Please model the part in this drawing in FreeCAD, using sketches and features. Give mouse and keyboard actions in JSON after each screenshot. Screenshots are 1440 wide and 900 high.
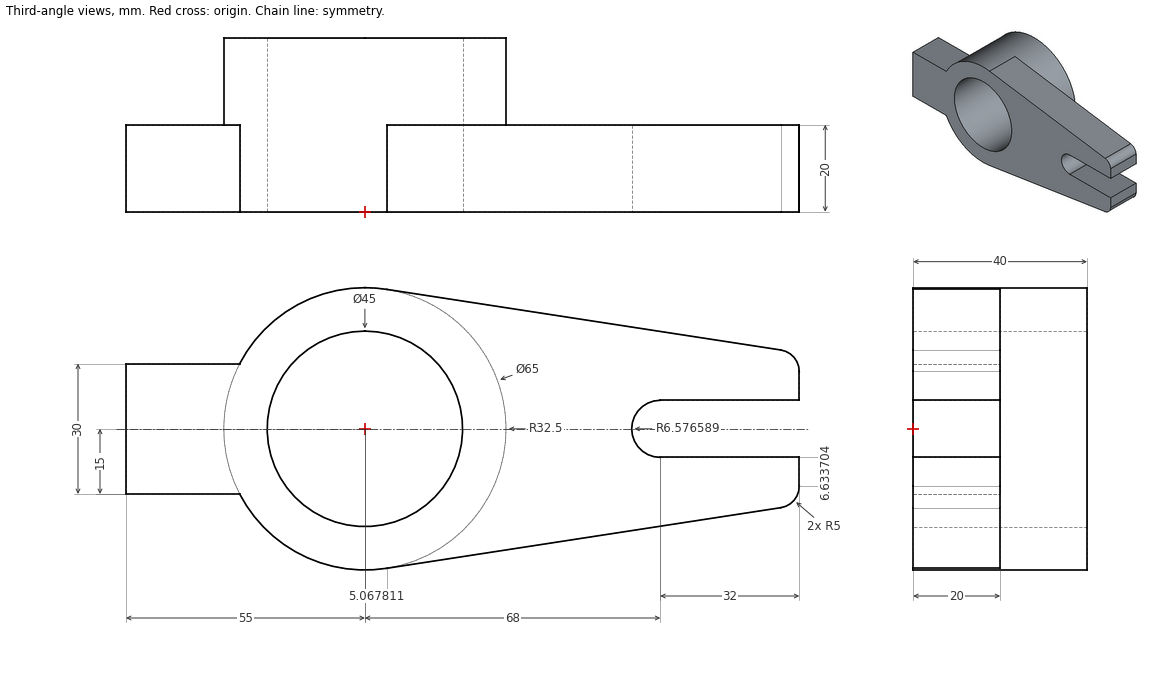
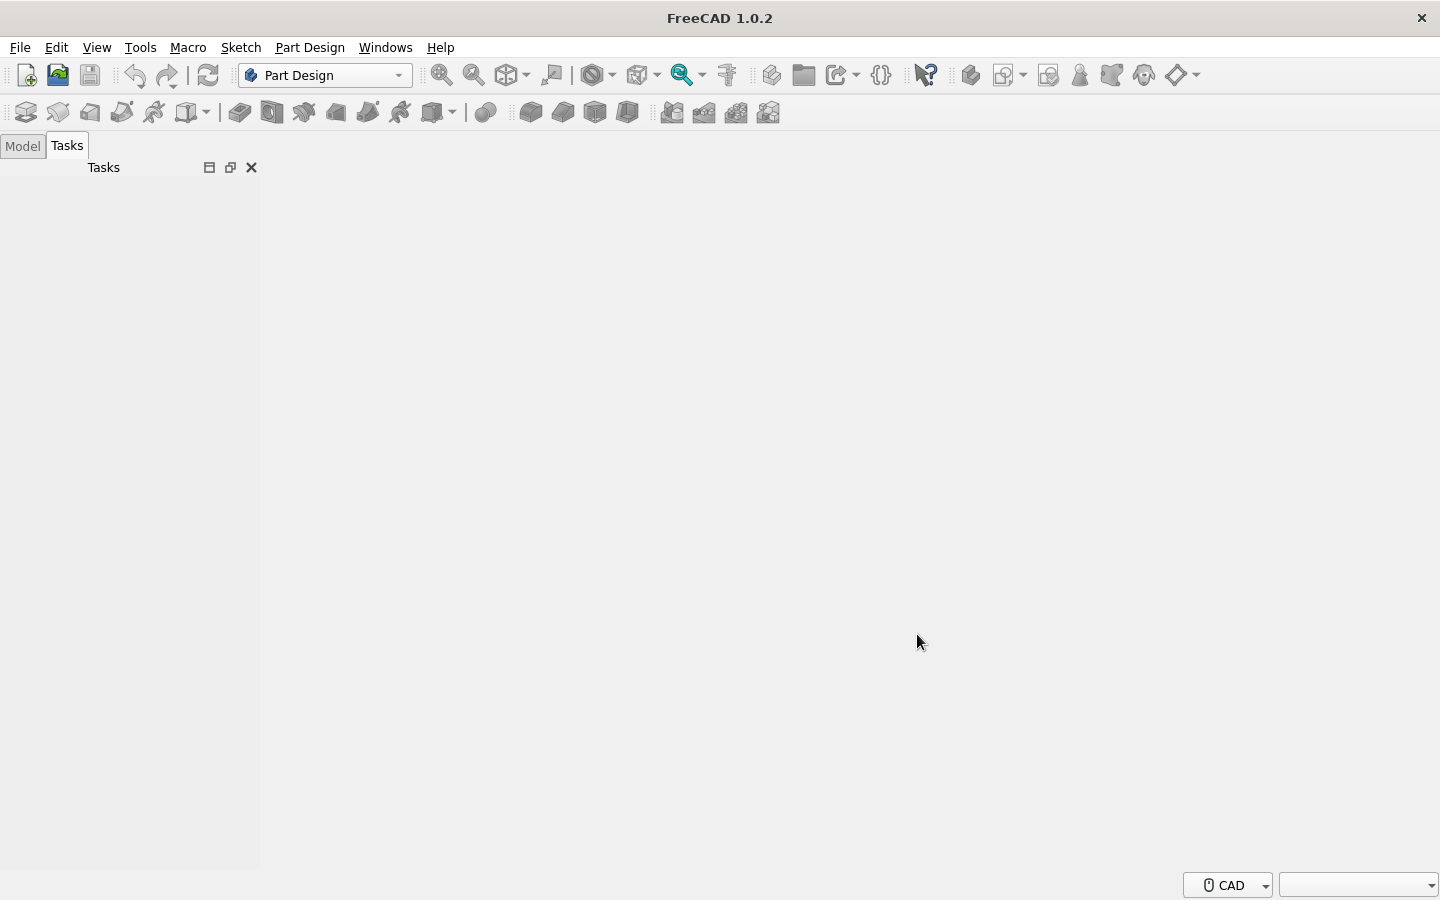
{"action": "left_click", "coordinate": [26, 76]}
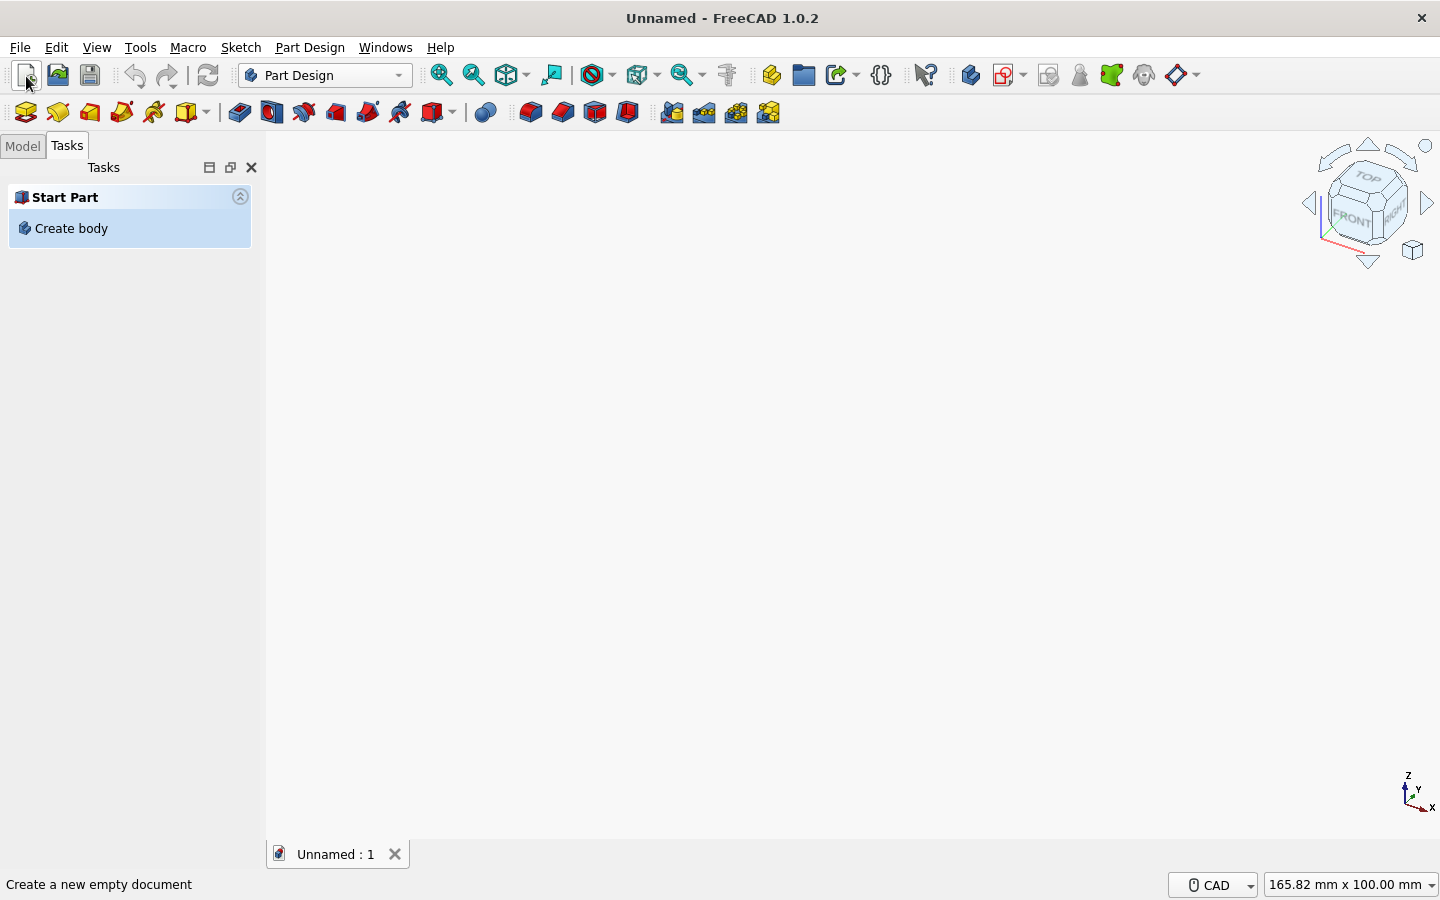
{"action": "left_click", "coordinate": [1004, 76]}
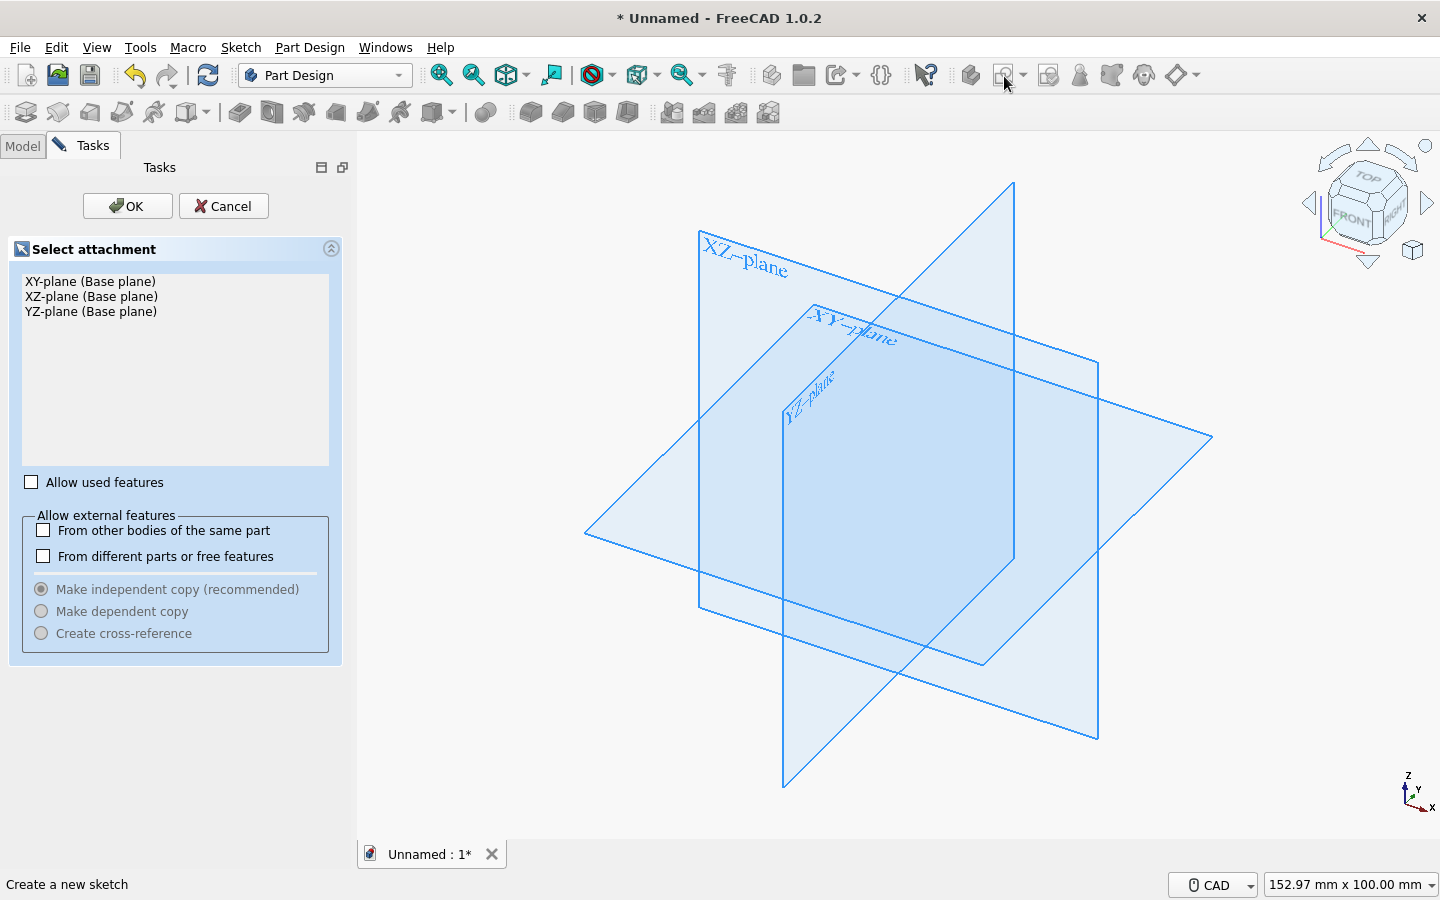
{"action": "left_click", "coordinate": [82, 296]}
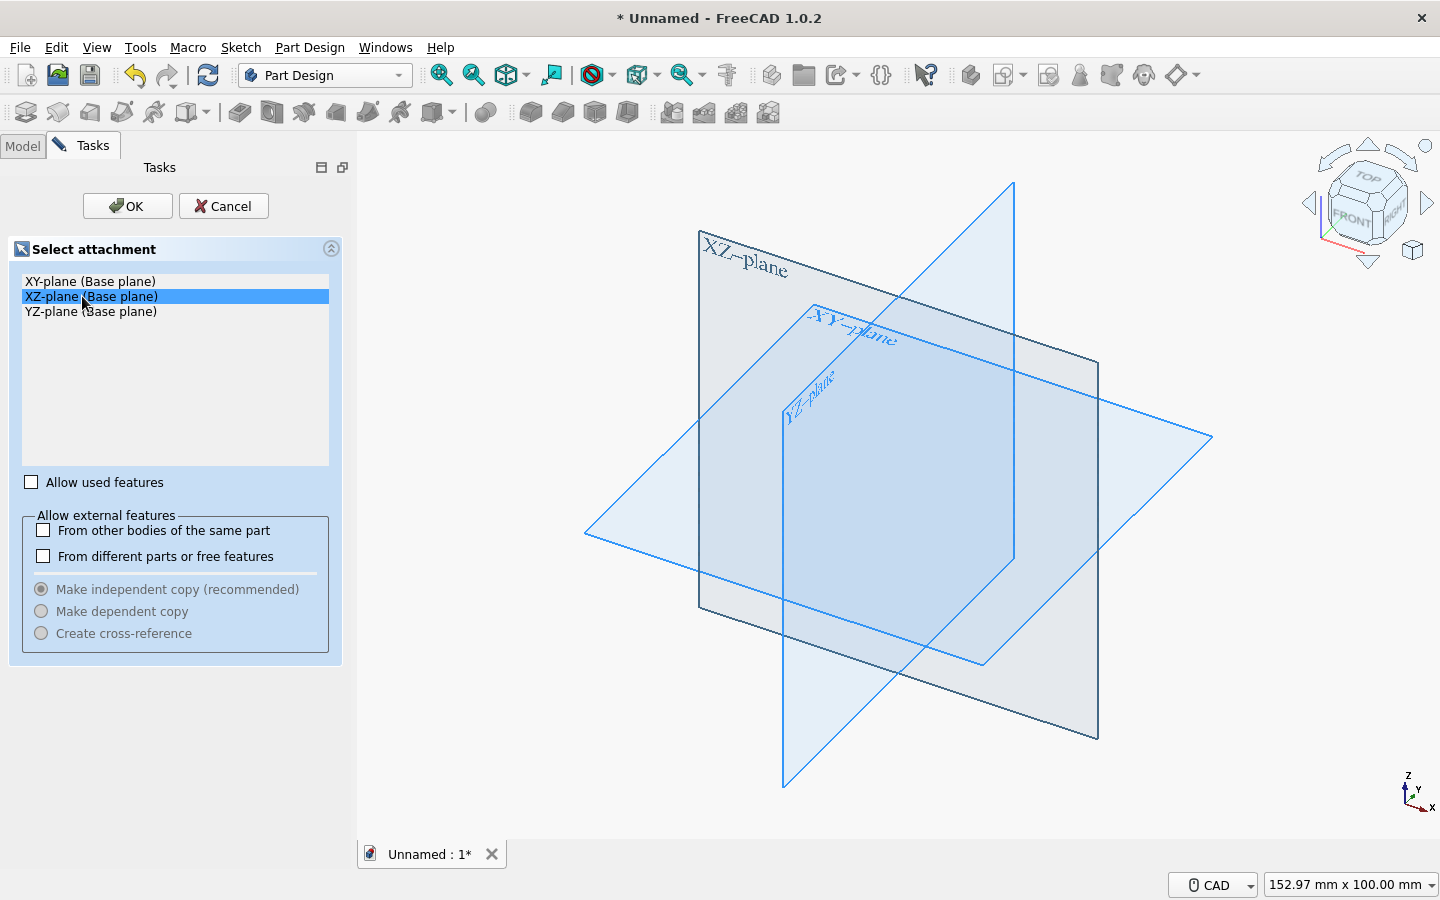
{"action": "left_click", "coordinate": [128, 206]}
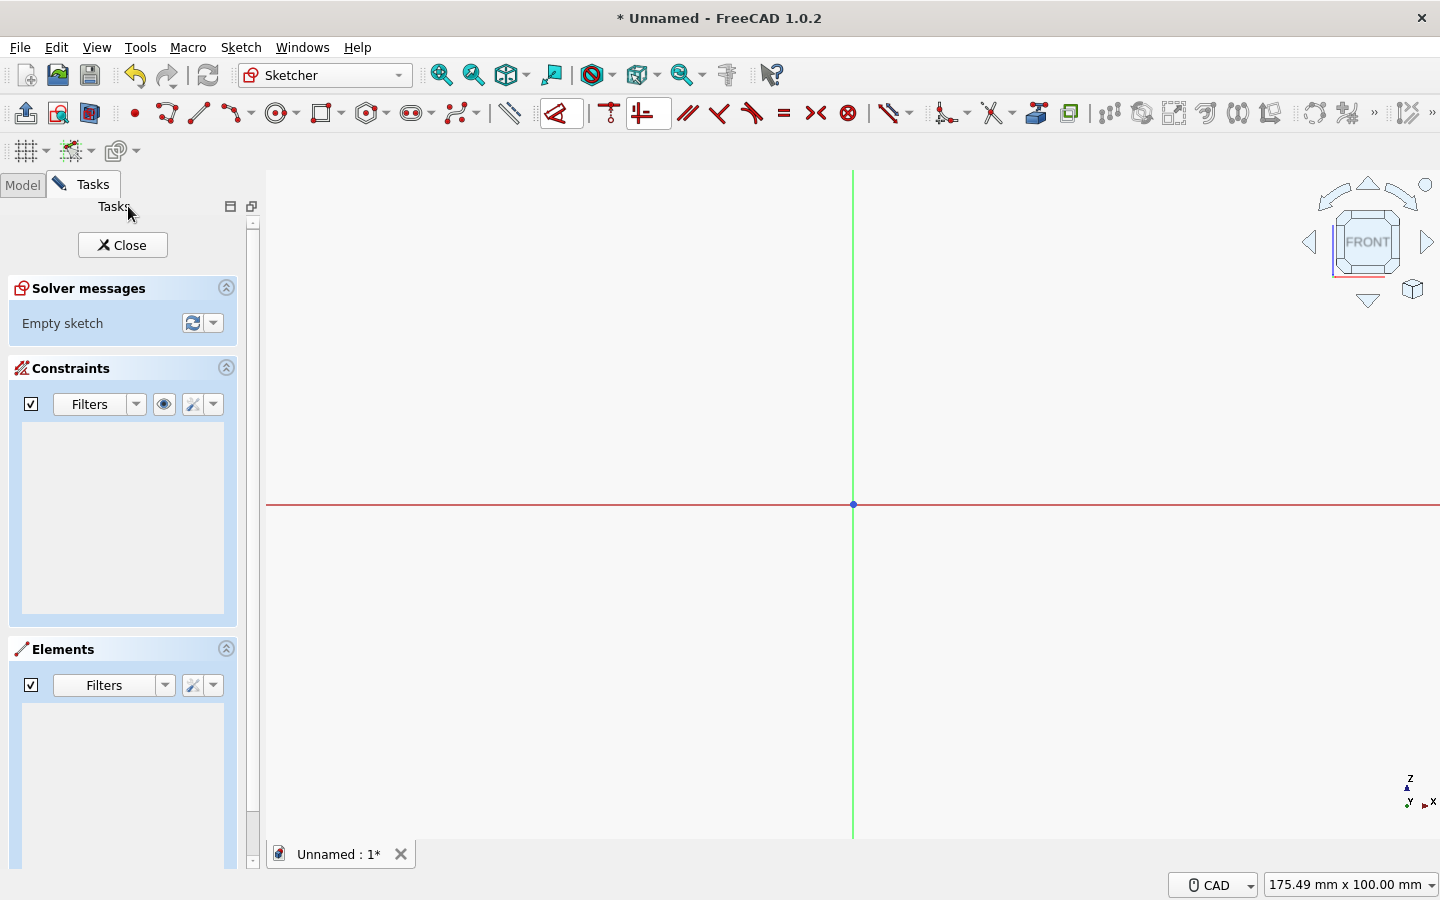
{"action": "left_click", "coordinate": [276, 114]}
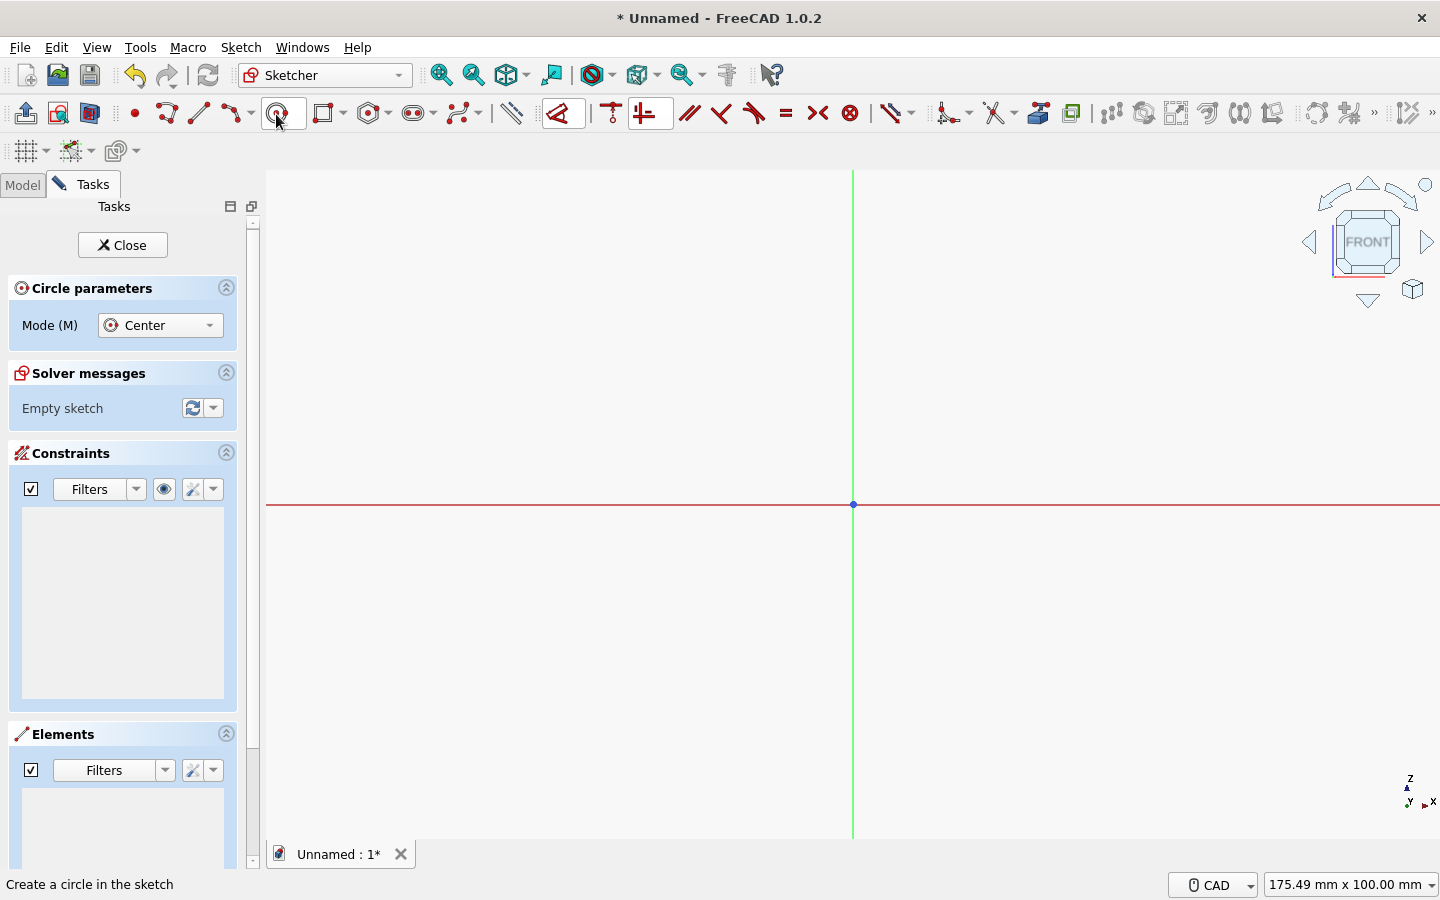
{"action": "left_click", "coordinate": [853, 504]}
{"action": "mouse_move", "coordinate": [1007, 351]}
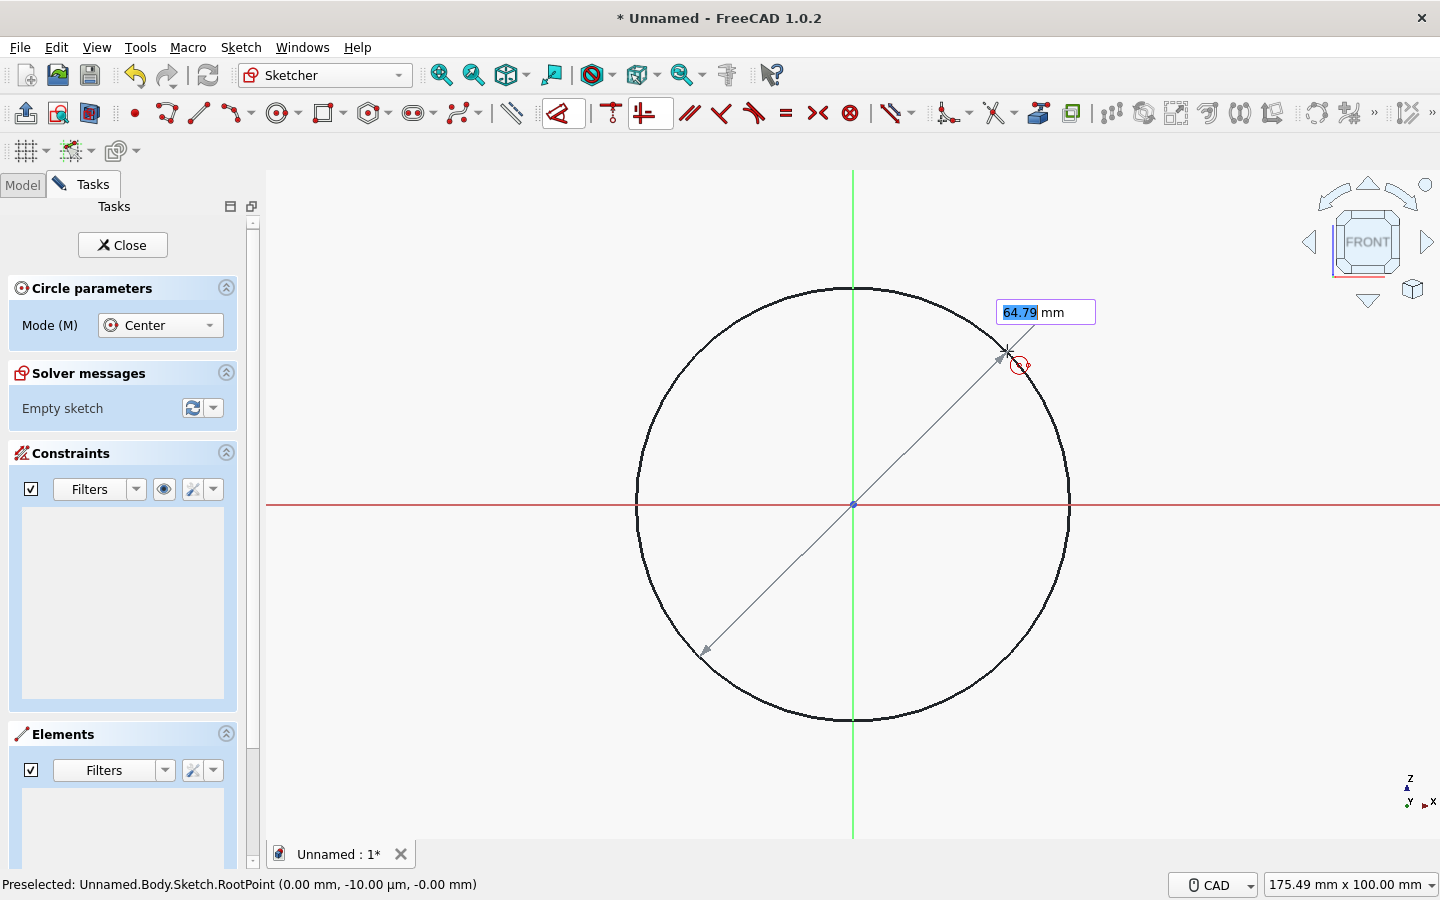
{"action": "type", "text": "65"}
{"action": "key", "text": "Return"}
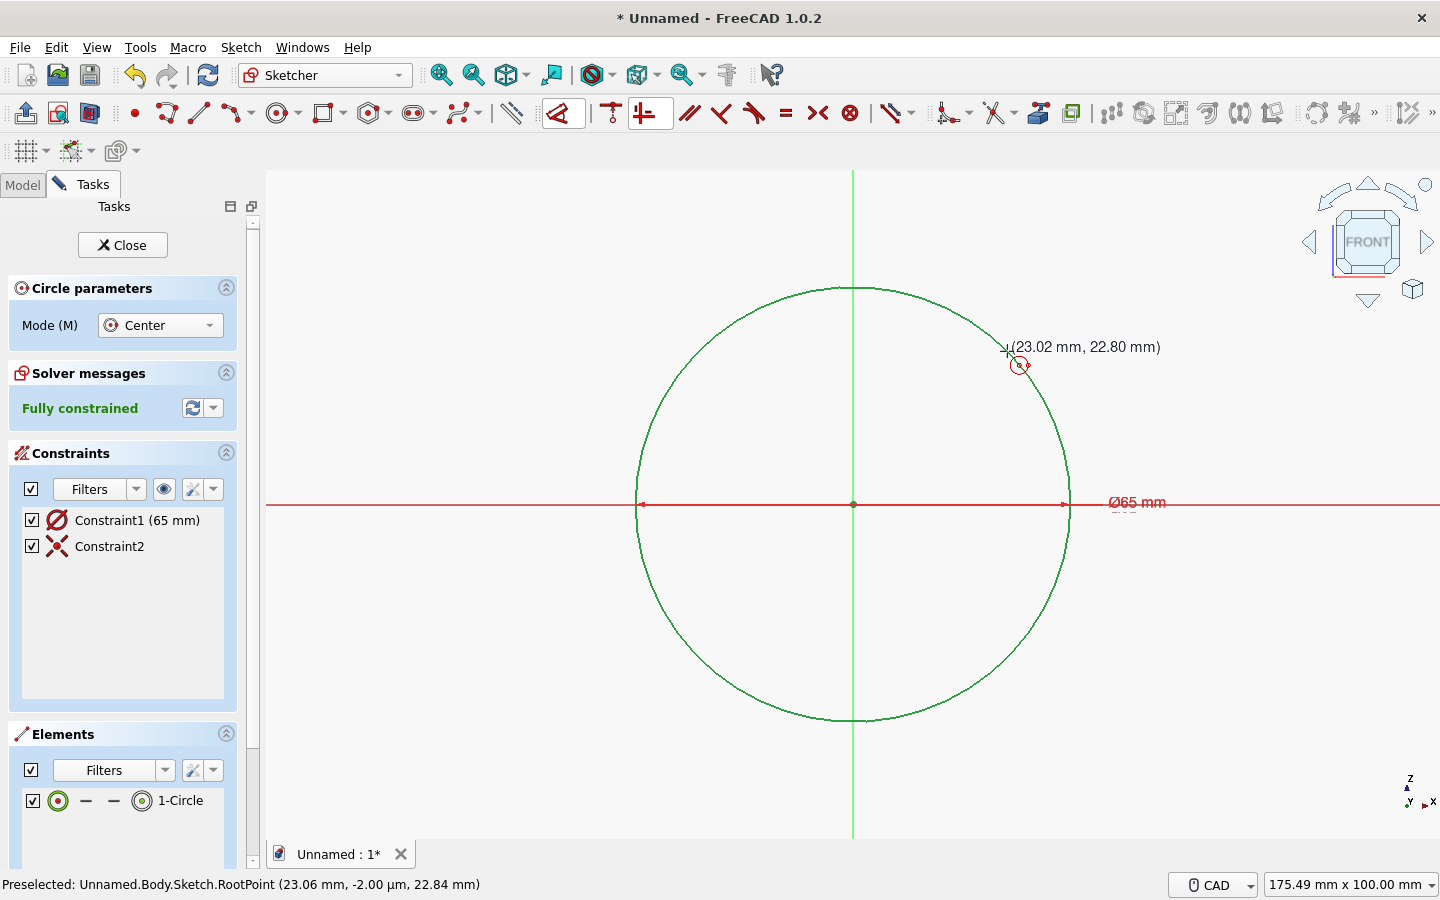
{"action": "left_click", "coordinate": [853, 504]}
{"action": "mouse_move", "coordinate": [959, 398]}